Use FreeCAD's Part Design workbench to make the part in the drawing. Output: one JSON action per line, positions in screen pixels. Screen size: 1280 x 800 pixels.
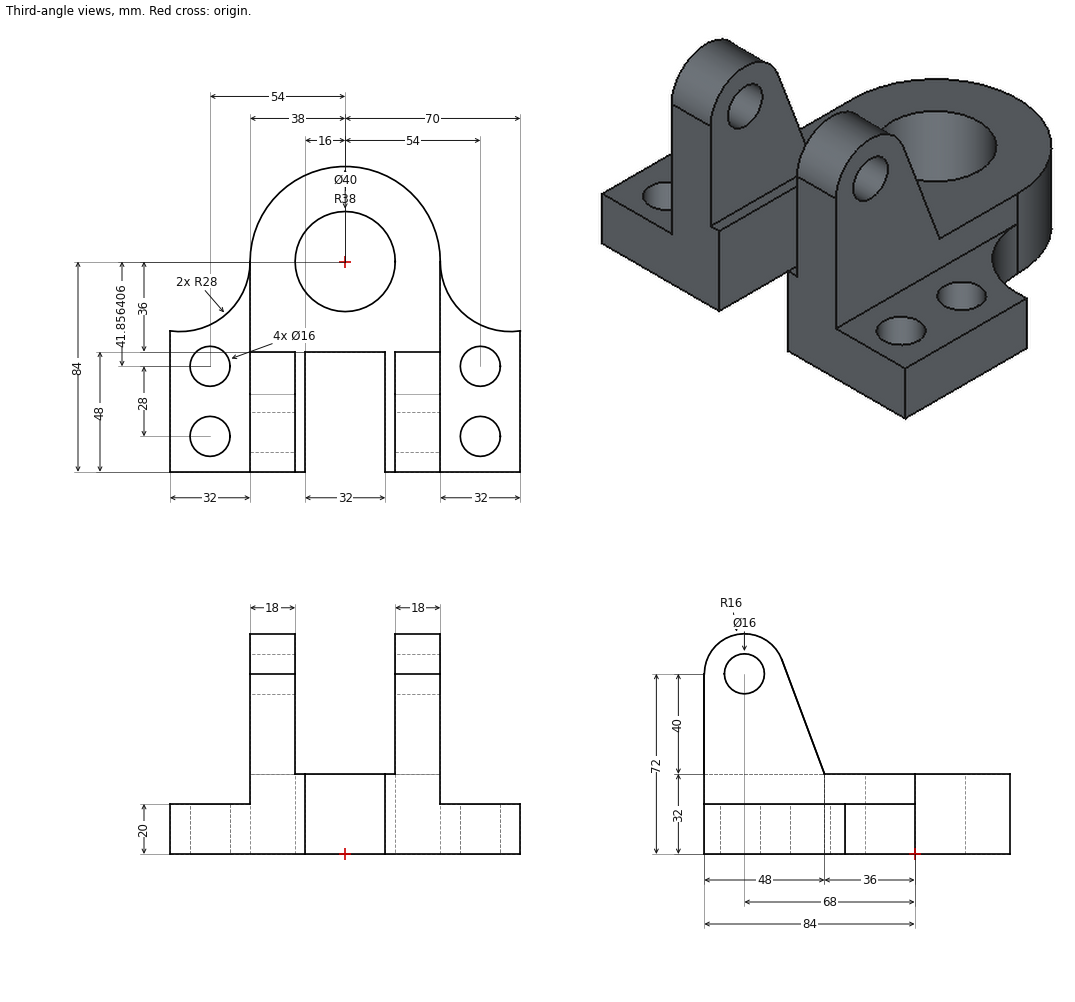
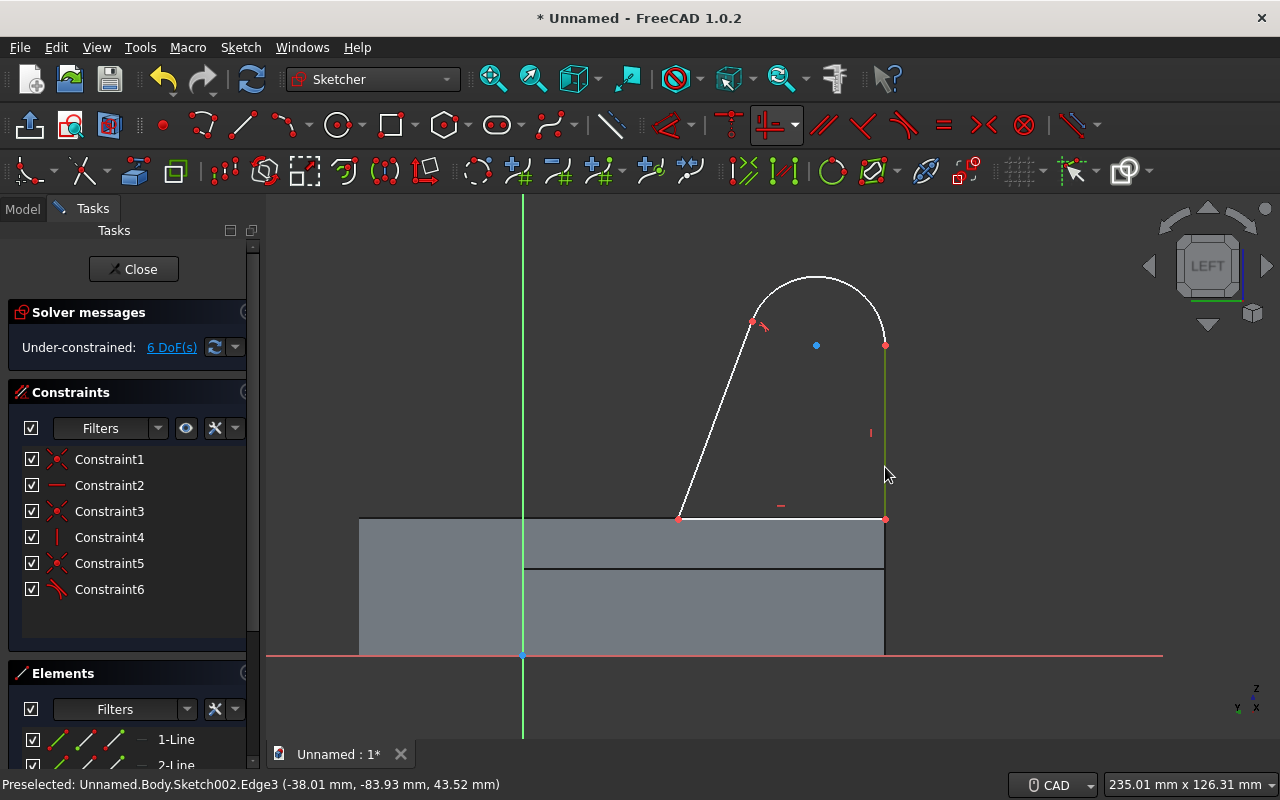
{"action": "left_click", "coordinate": [863, 295]}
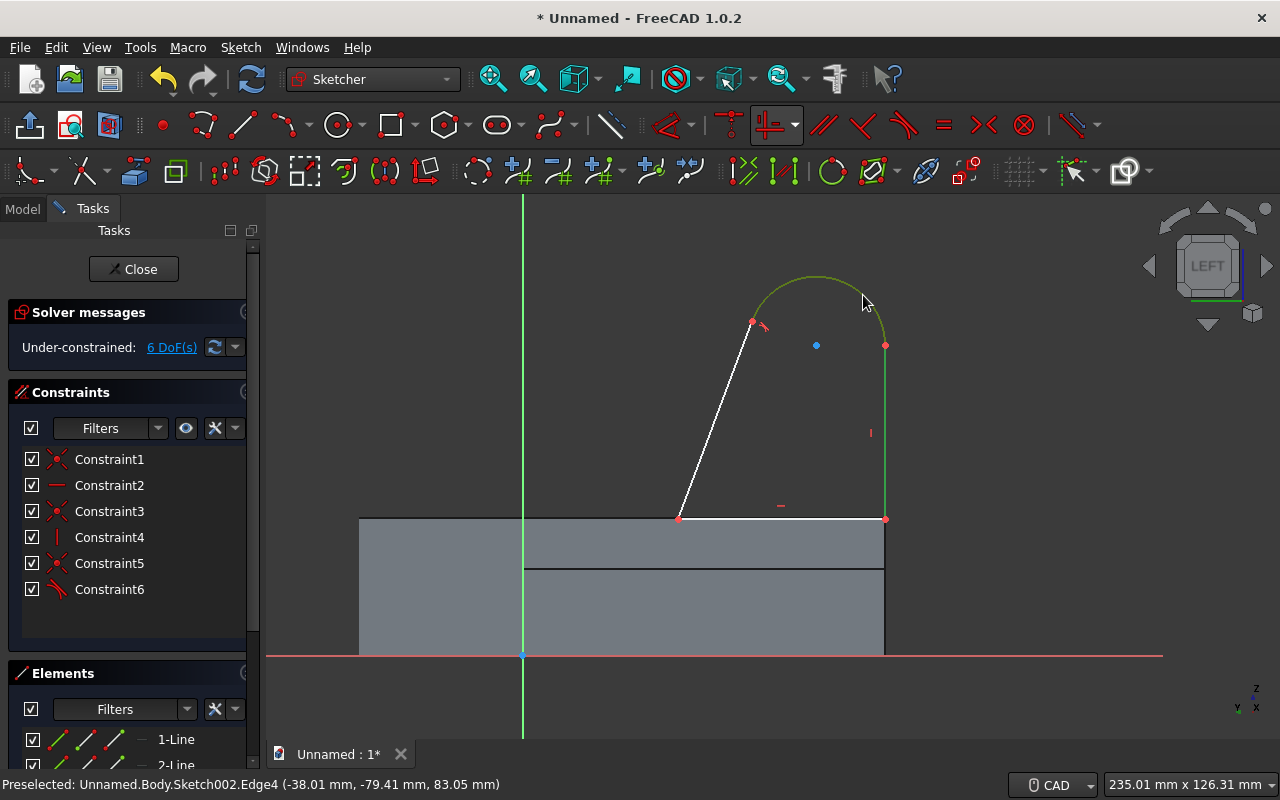
{"action": "left_click", "coordinate": [904, 126]}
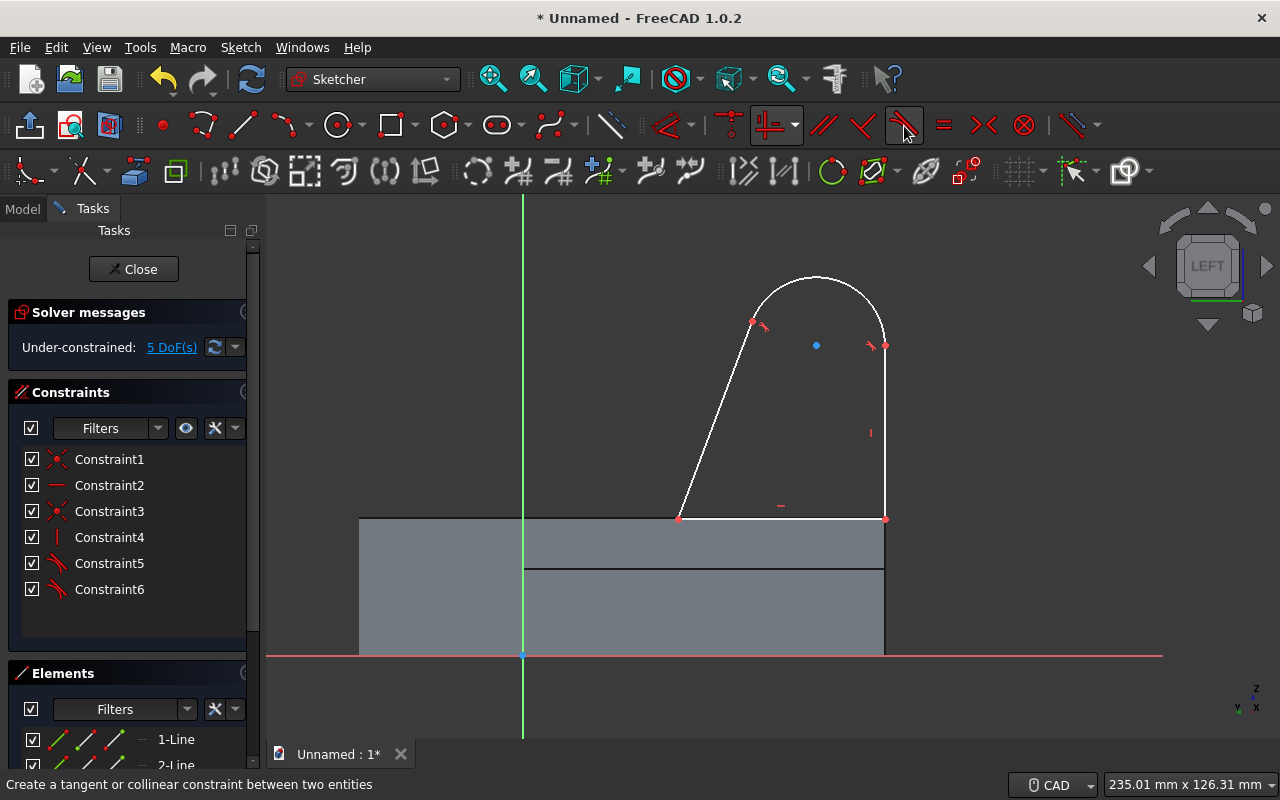
{"action": "left_click", "coordinate": [666, 126]}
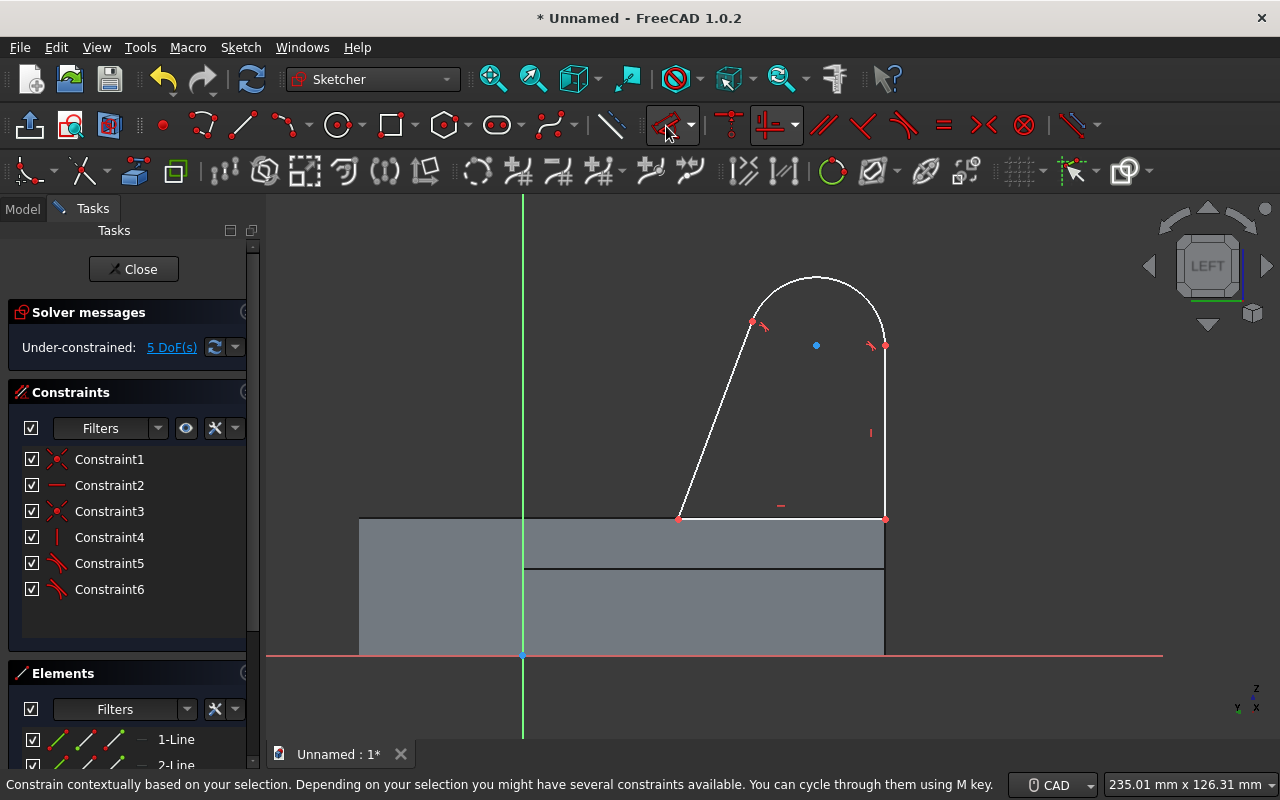
{"action": "left_click", "coordinate": [862, 295]}
{"action": "left_click", "coordinate": [883, 271]}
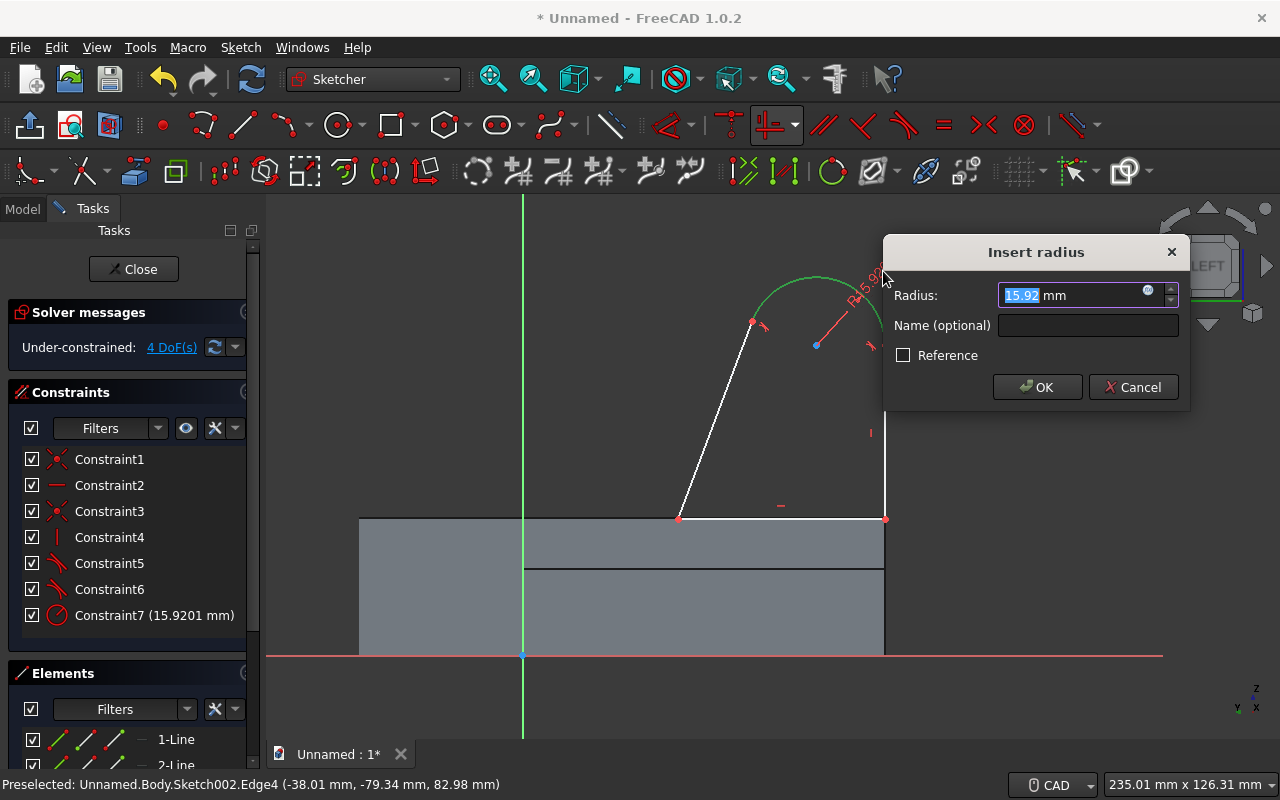
{"action": "type", "text": "16"}
{"action": "key", "text": "Return"}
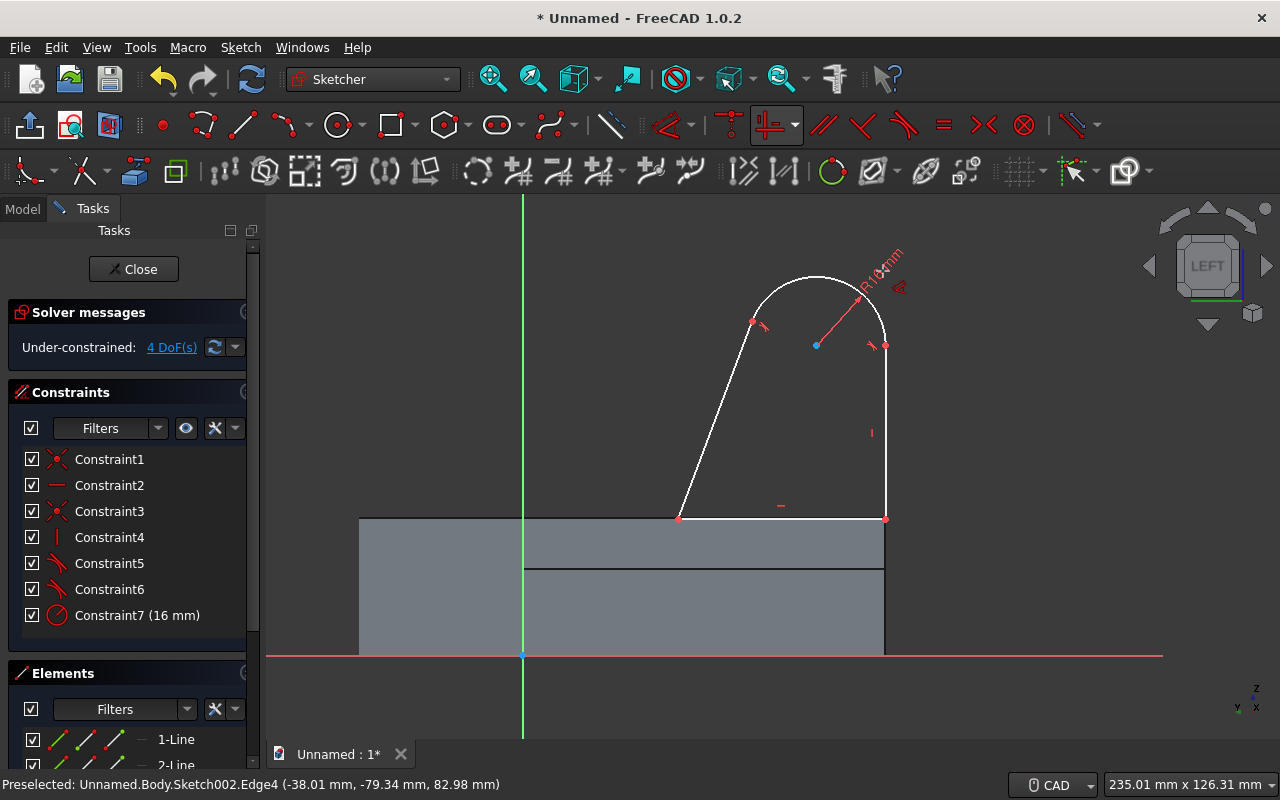
{"action": "left_click", "coordinate": [740, 519]}
{"action": "left_click", "coordinate": [782, 553]}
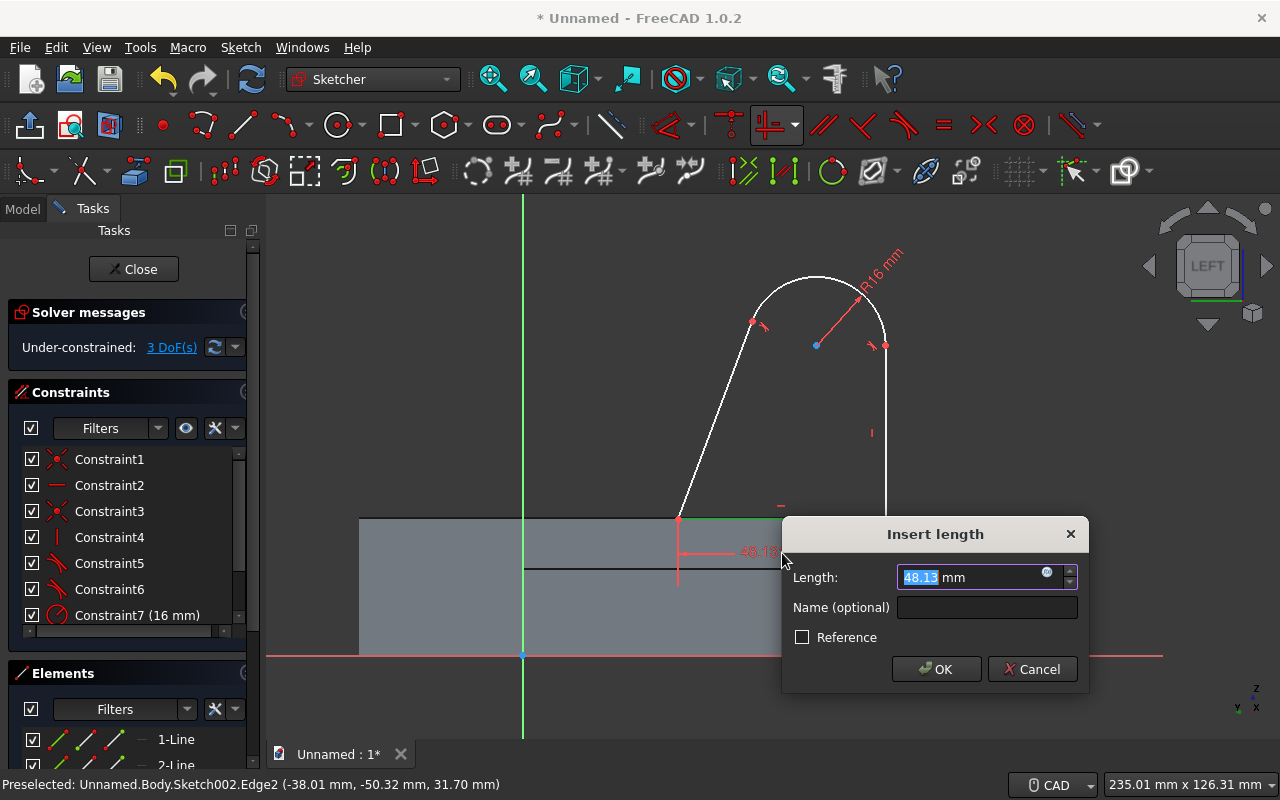
{"action": "type", "text": "48"}
{"action": "key", "text": "Return"}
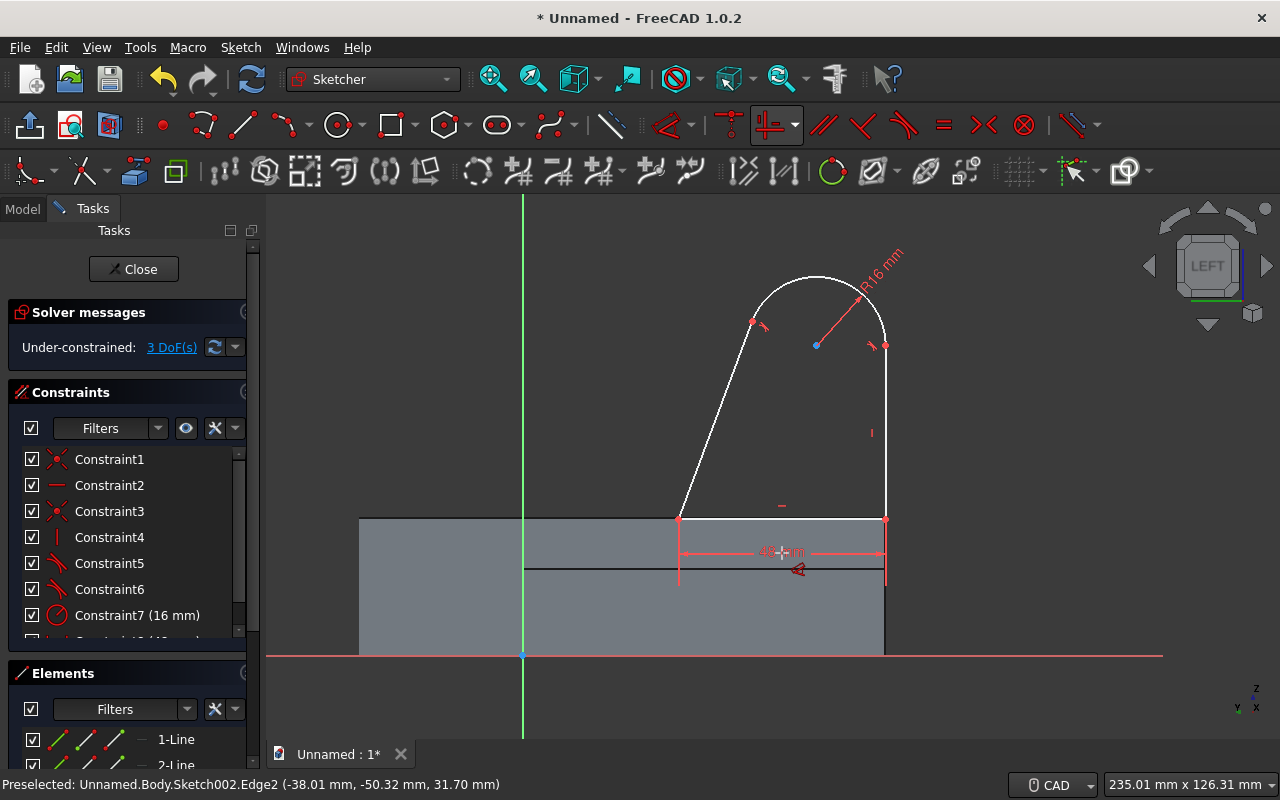
{"action": "left_click", "coordinate": [886, 467]}
{"action": "left_click", "coordinate": [920, 432]}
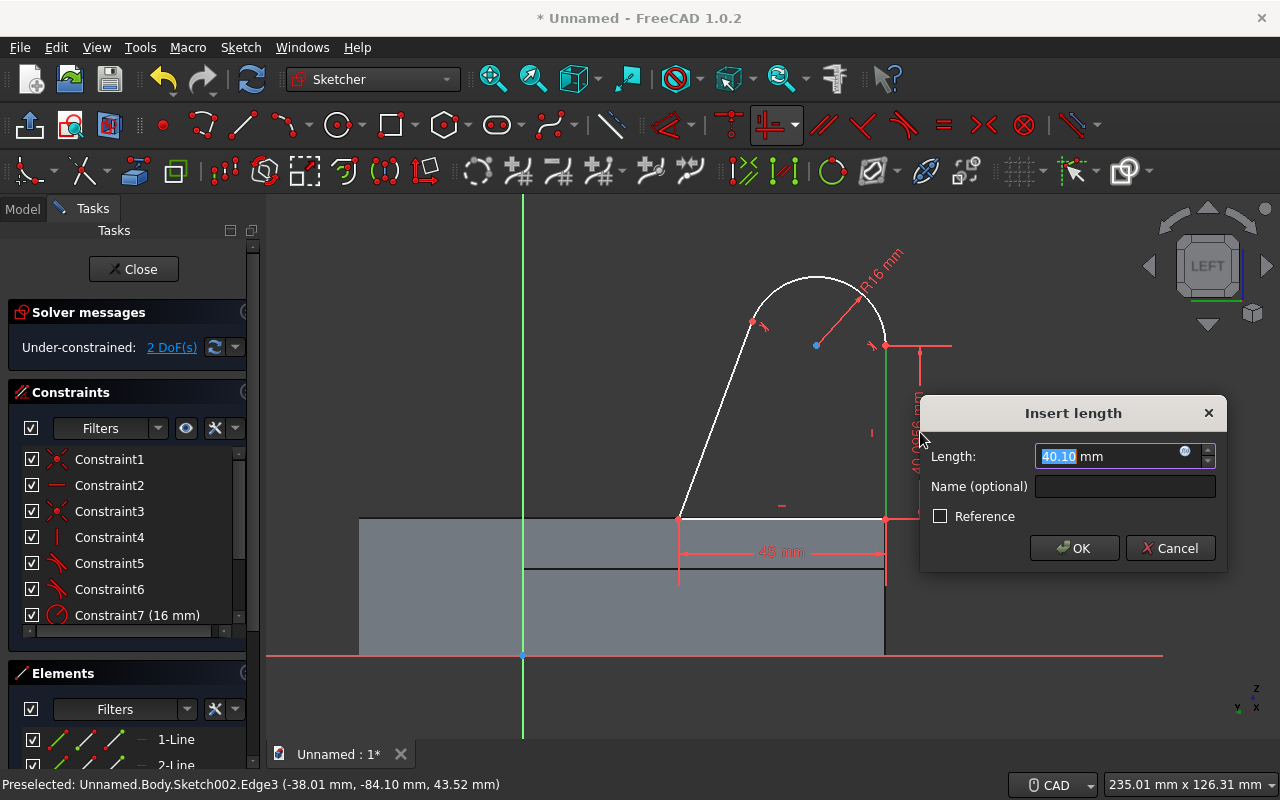
{"action": "type", "text": "40"}
{"action": "key", "text": "Return"}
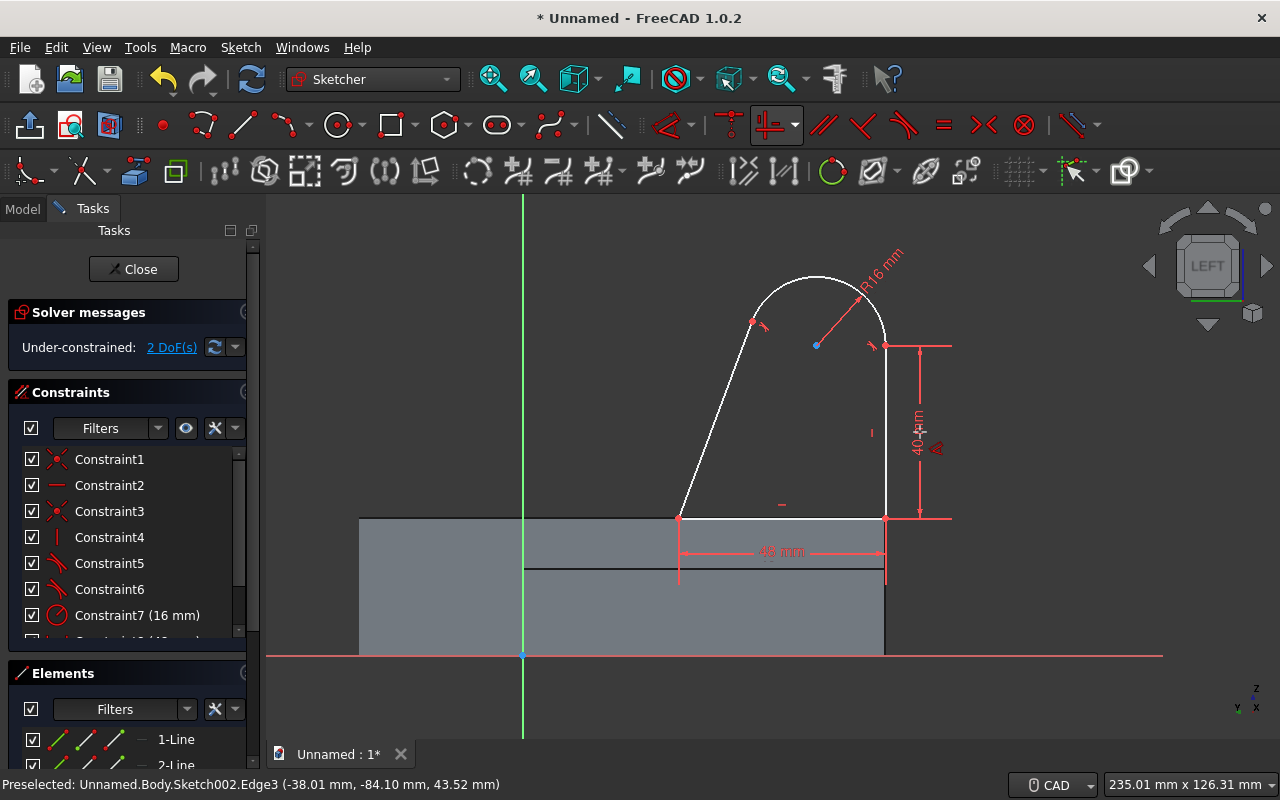
{"action": "left_click", "coordinate": [679, 519]}
{"action": "left_click", "coordinate": [601, 690]}